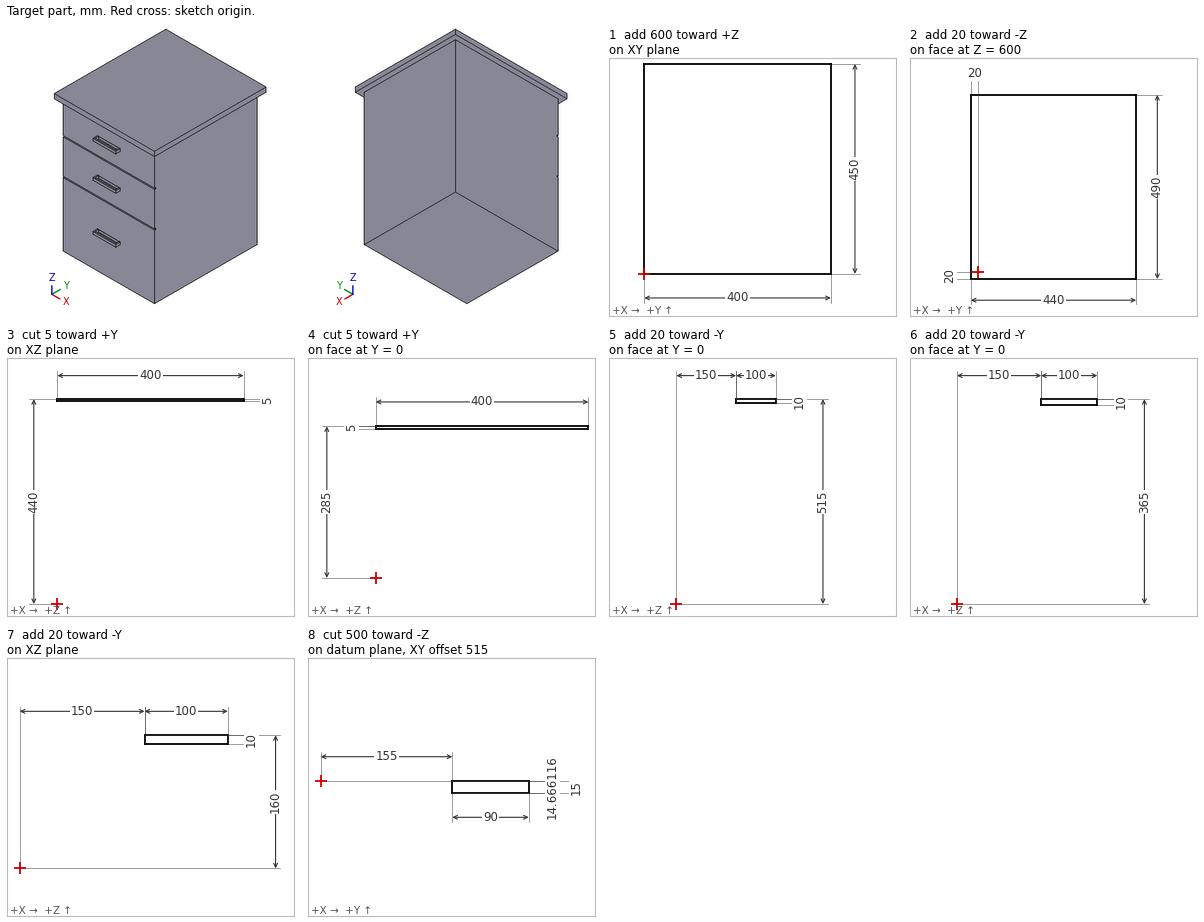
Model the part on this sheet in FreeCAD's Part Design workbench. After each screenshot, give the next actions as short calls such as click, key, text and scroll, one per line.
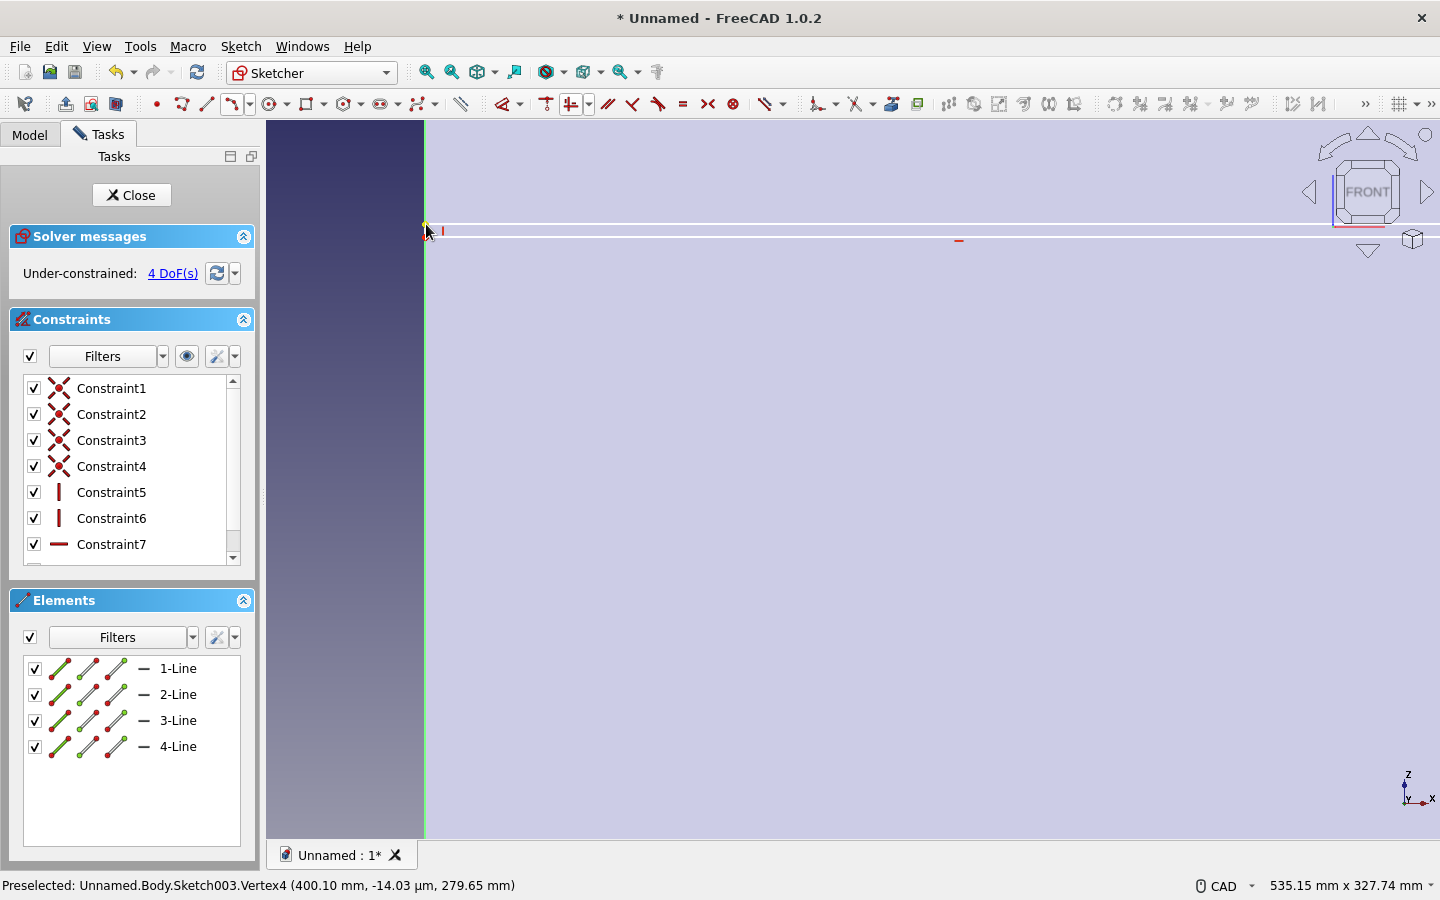
click(425, 224)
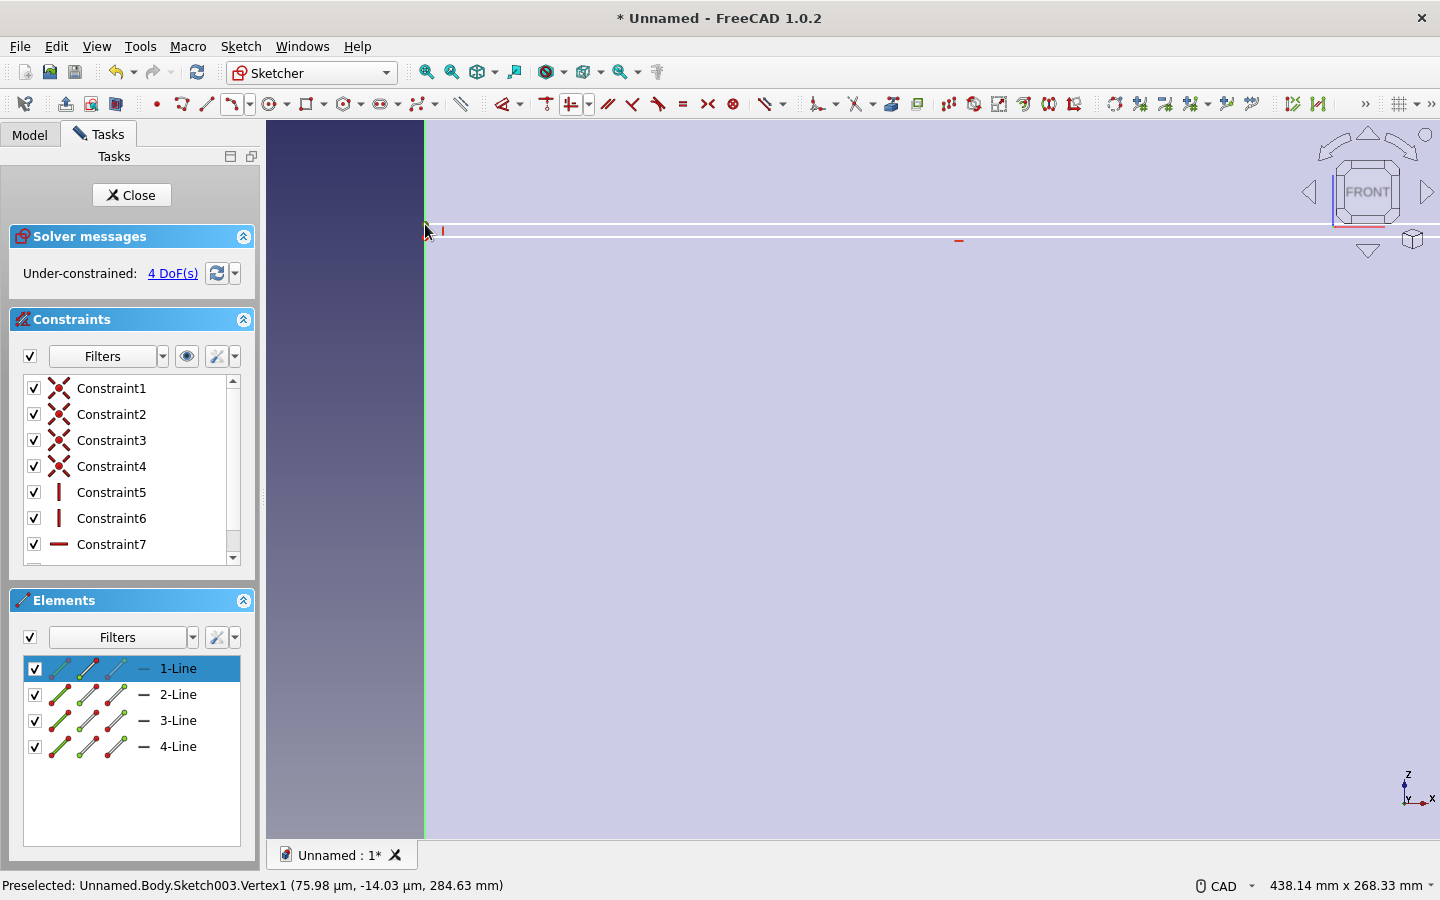
click(425, 764)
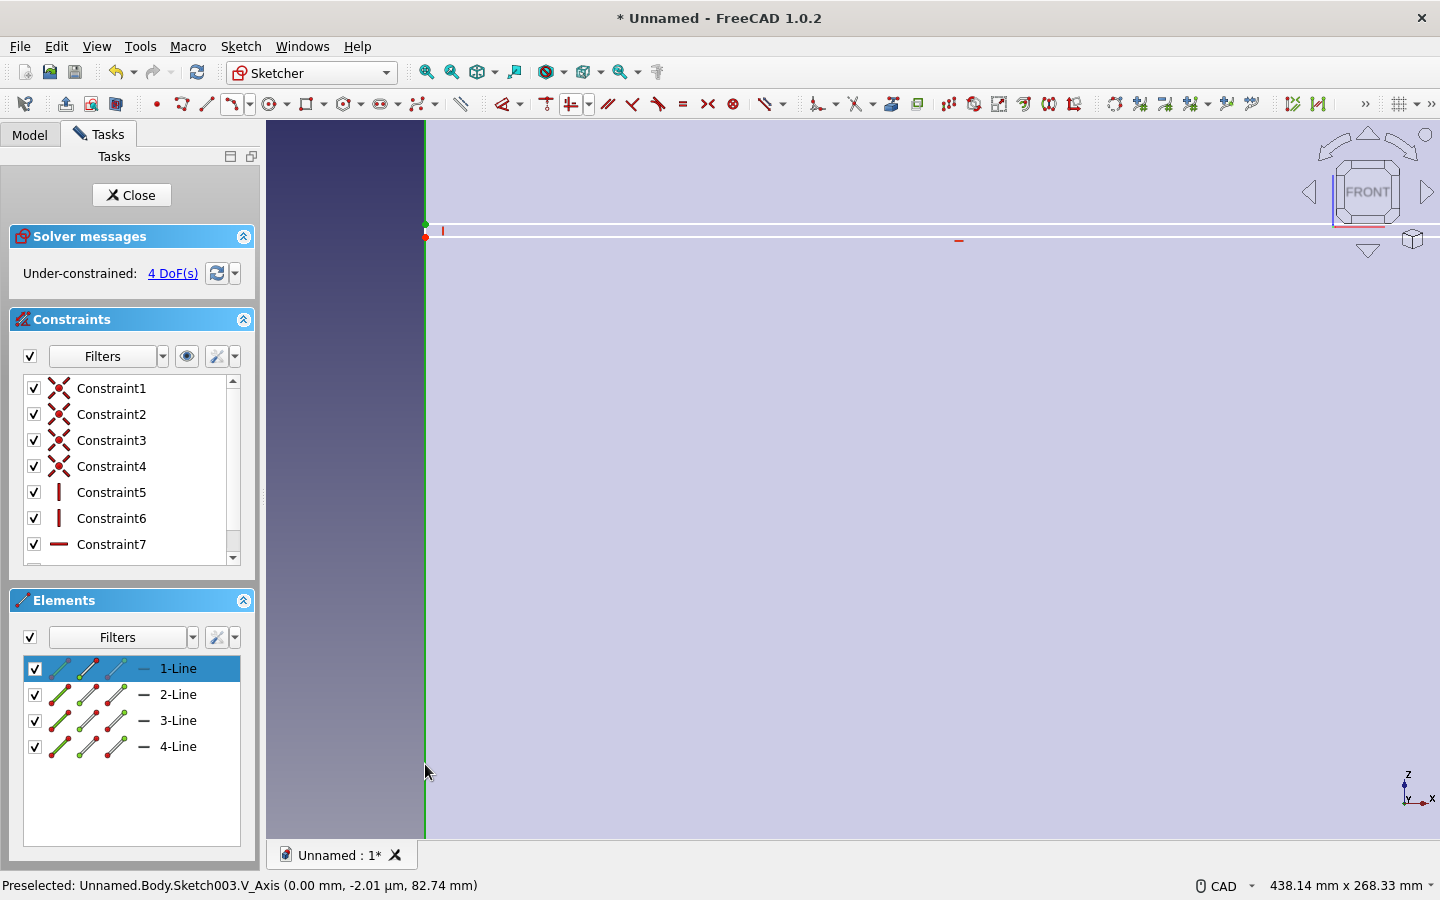
click(546, 104)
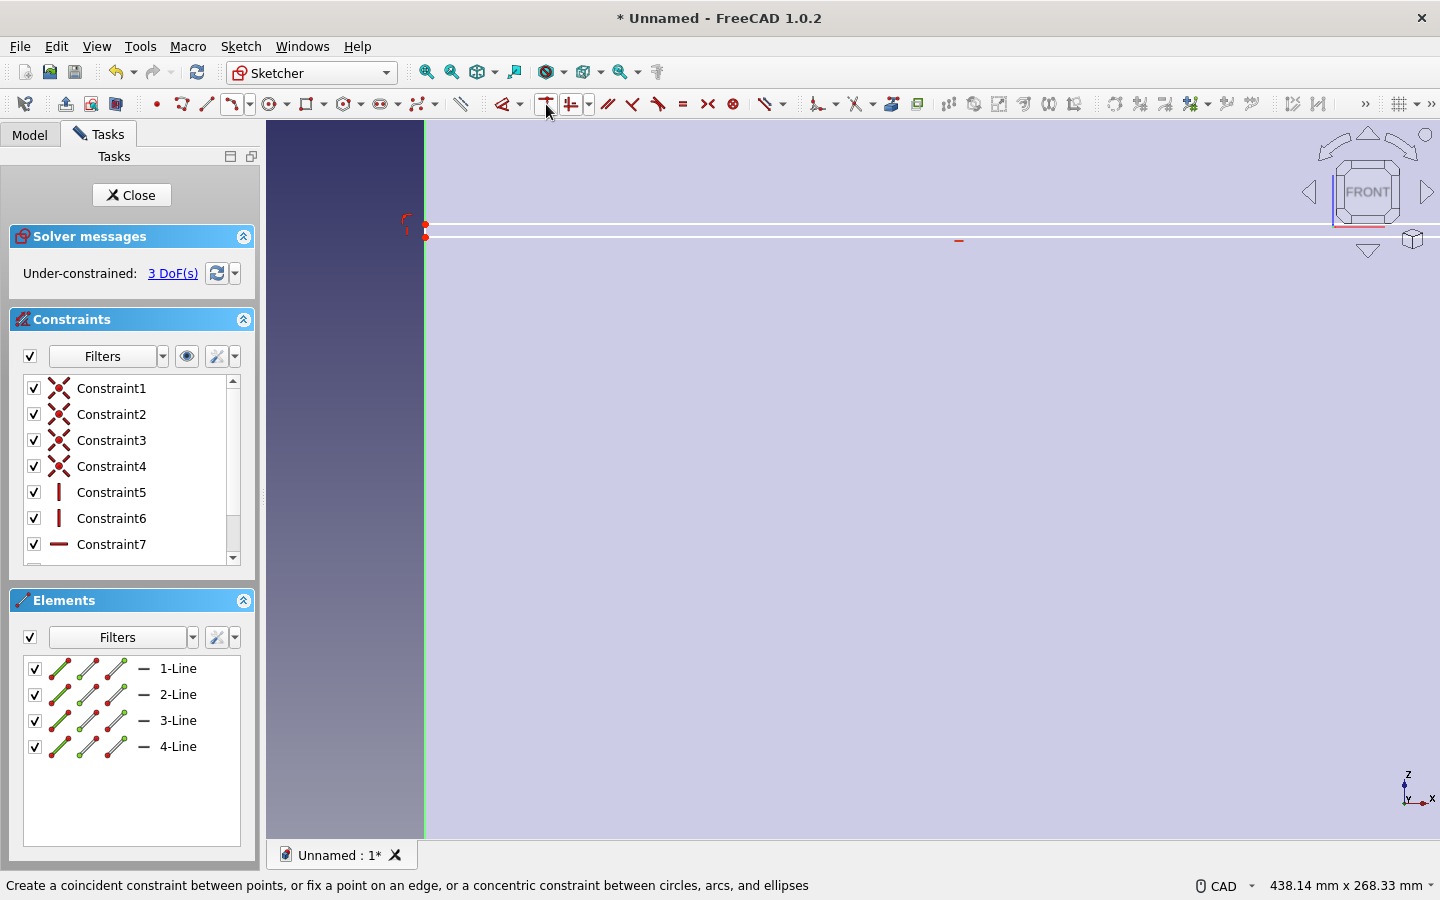
click(502, 104)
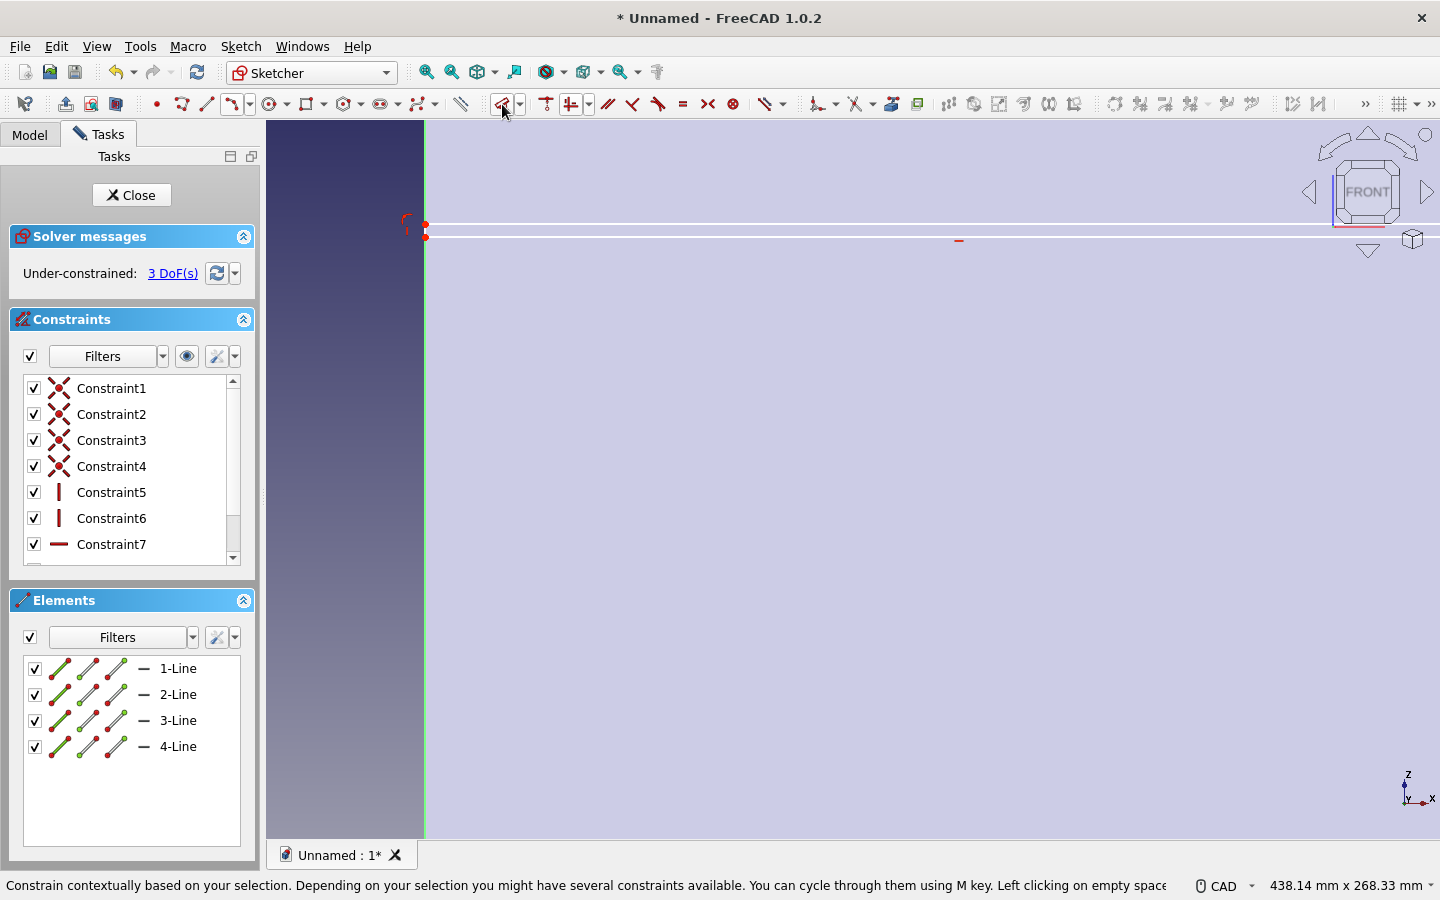
scroll(425, 231, up, 6)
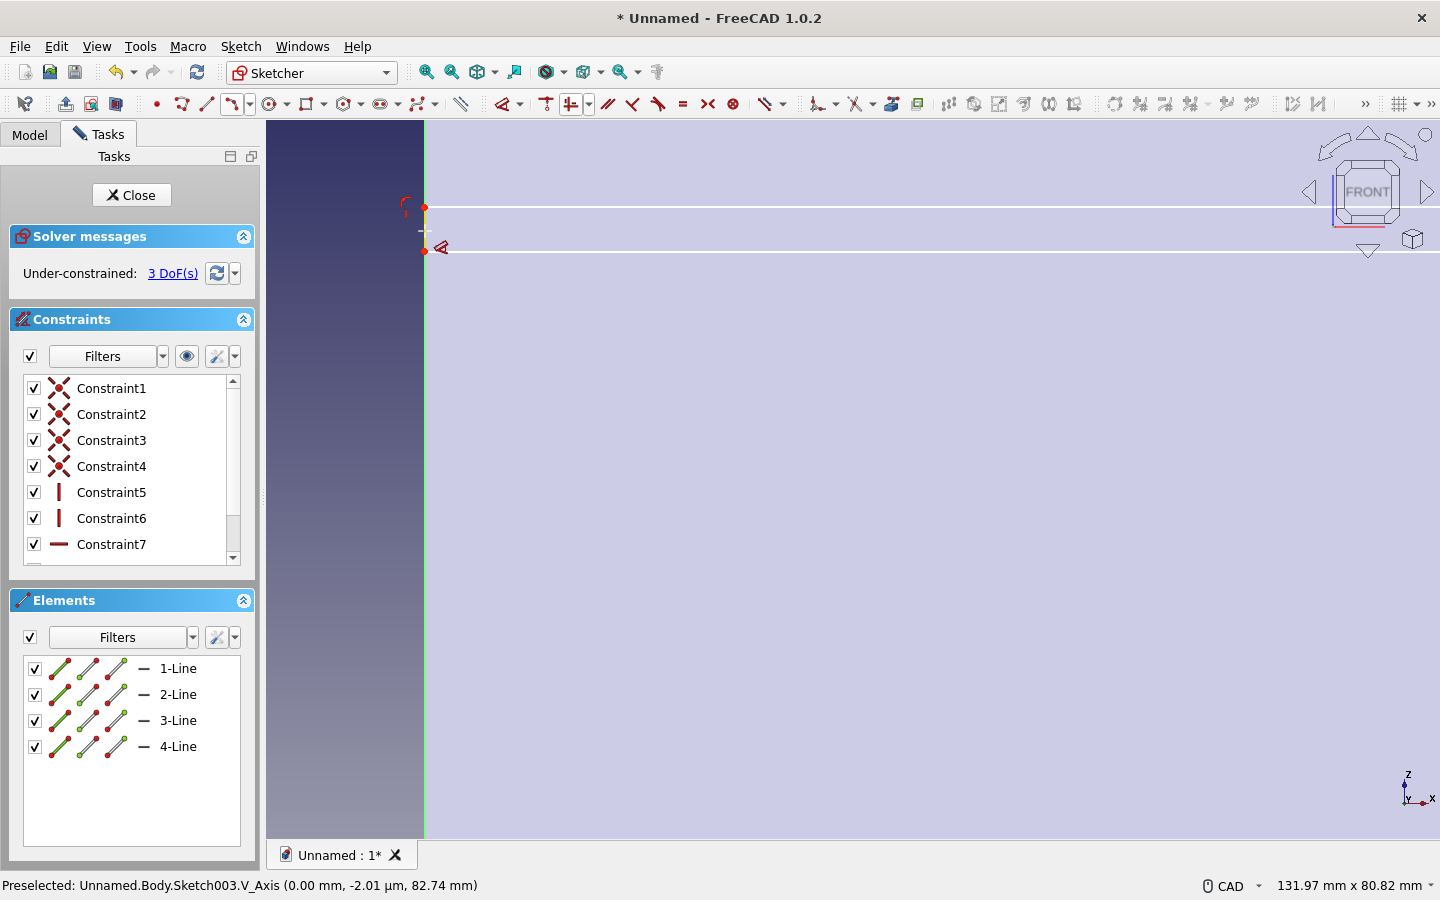
click(425, 230)
click(391, 230)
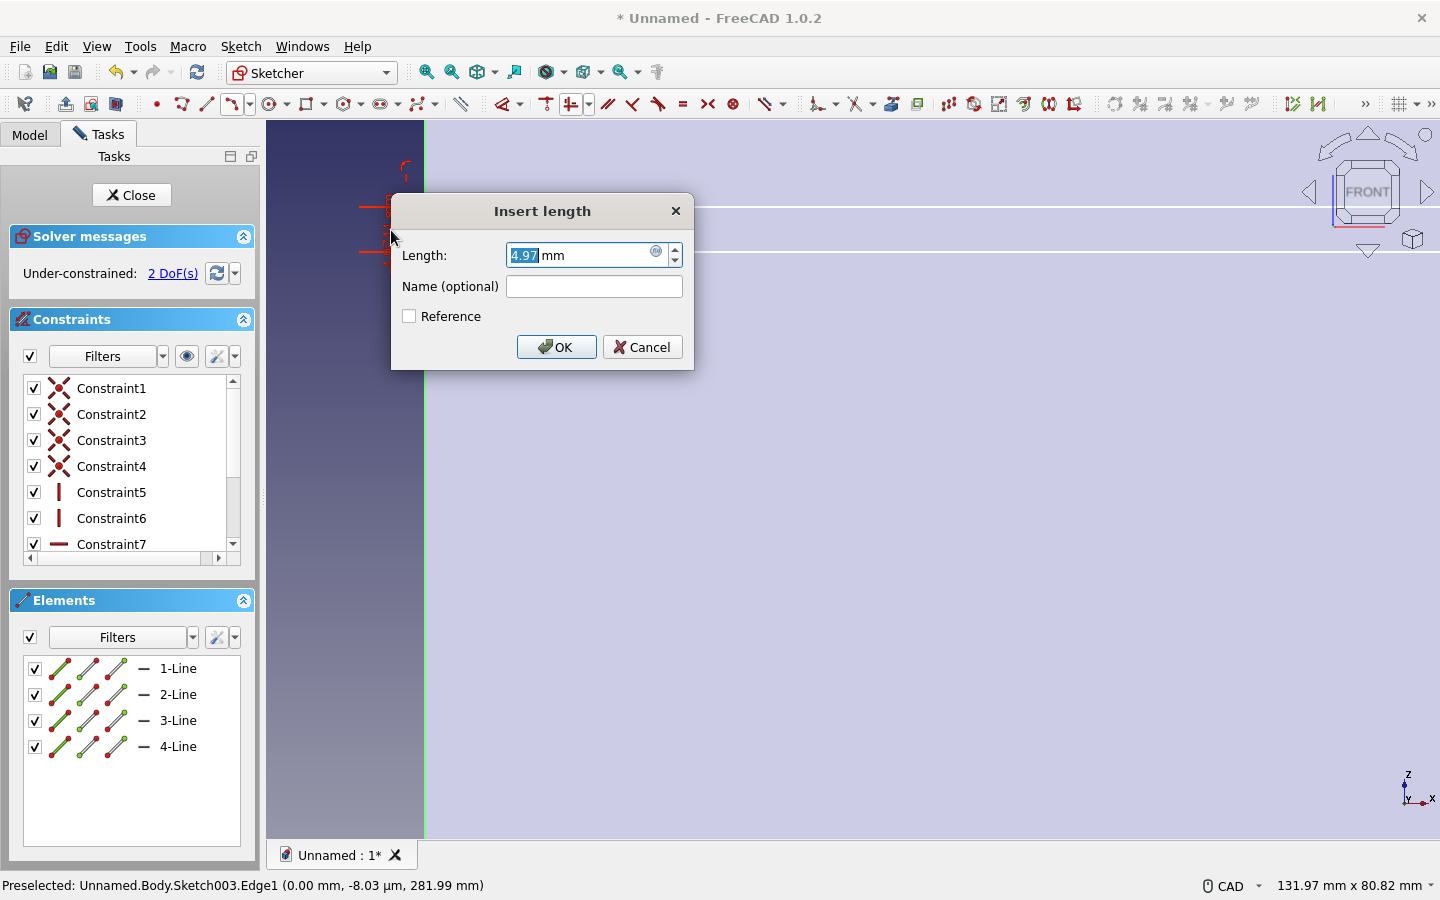
text(5)
key(Return)